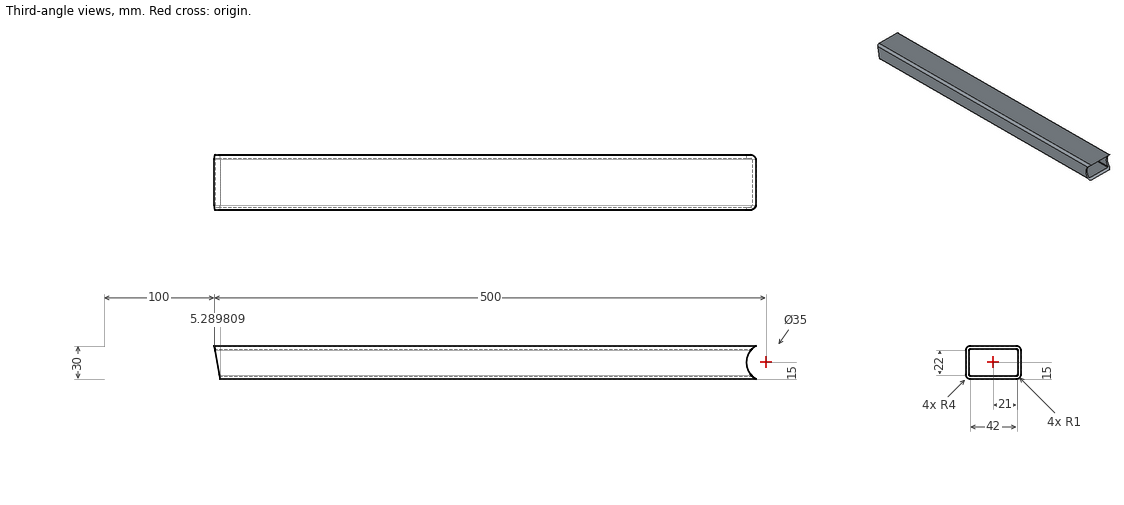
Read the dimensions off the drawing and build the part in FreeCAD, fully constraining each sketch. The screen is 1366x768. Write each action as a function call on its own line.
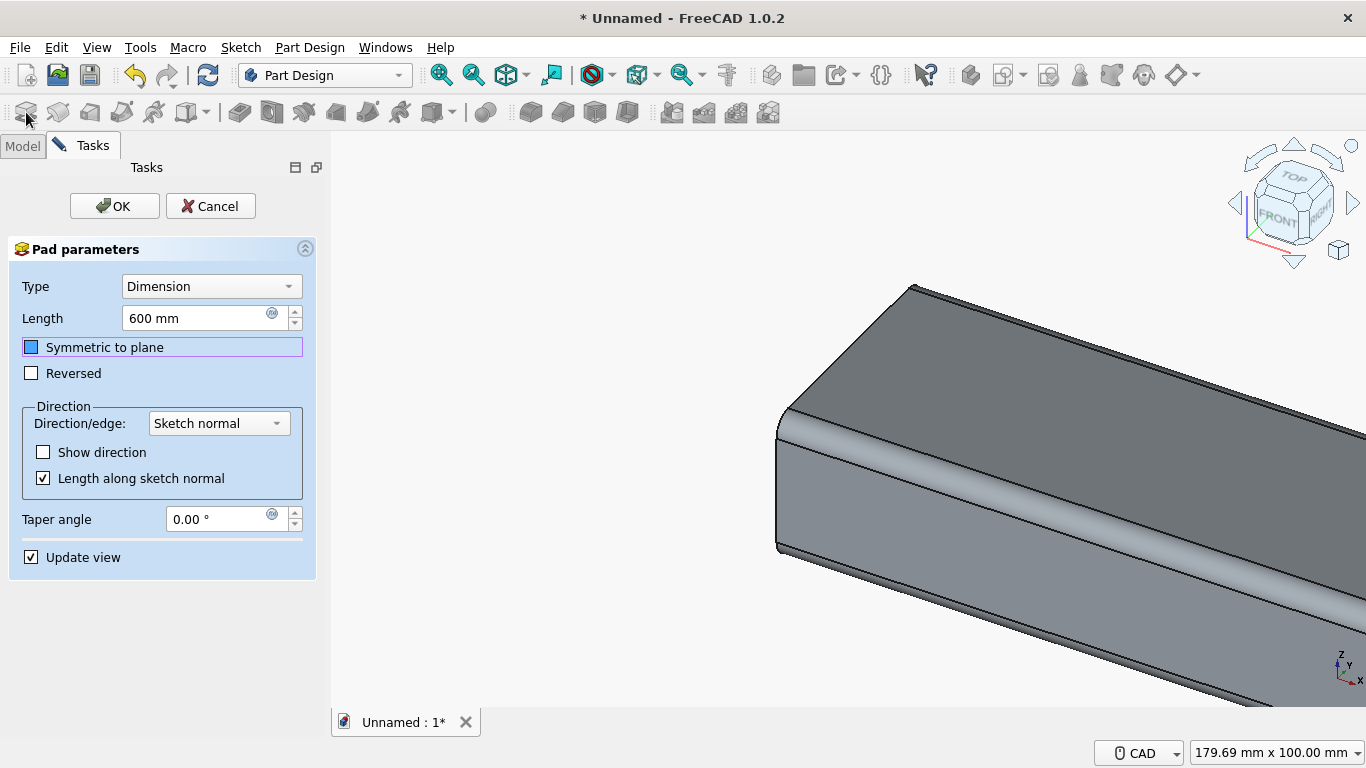
click(30, 373)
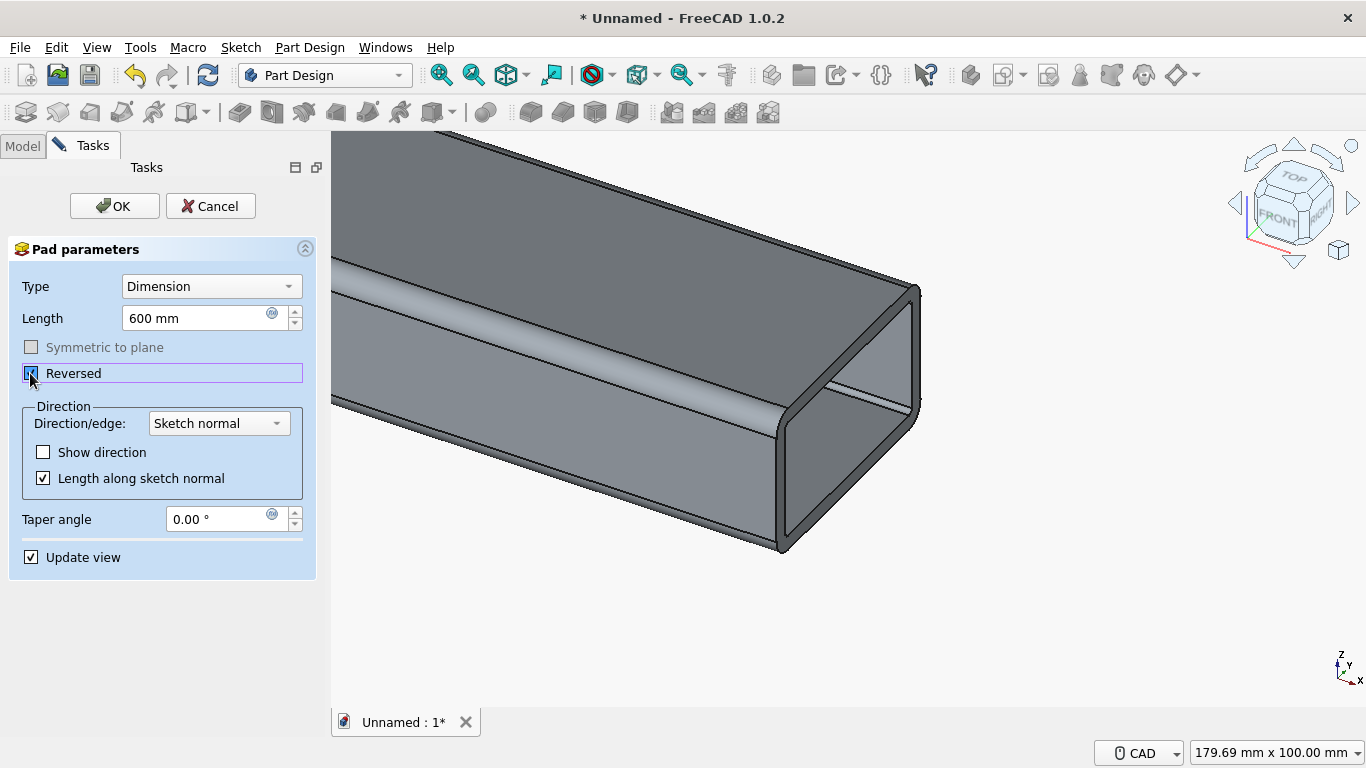
click(115, 206)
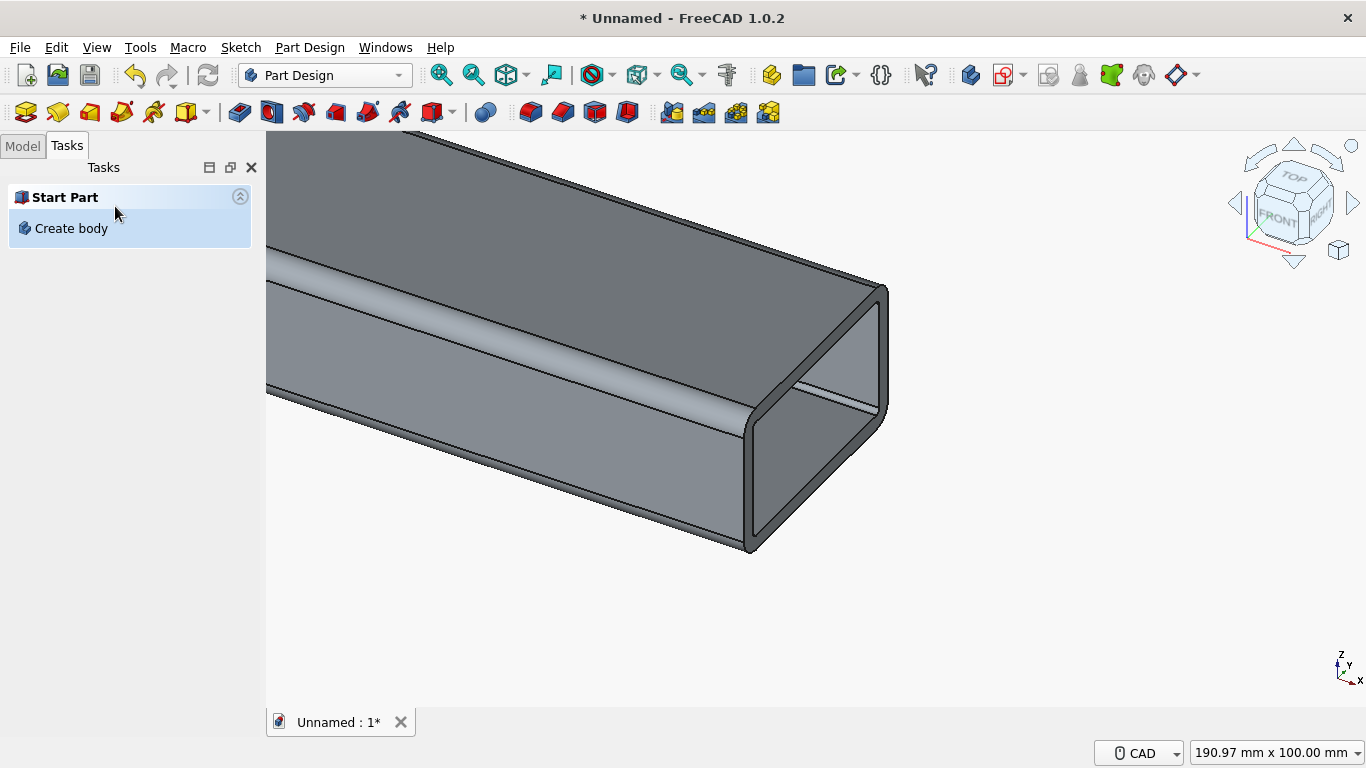
key(v)
key(f)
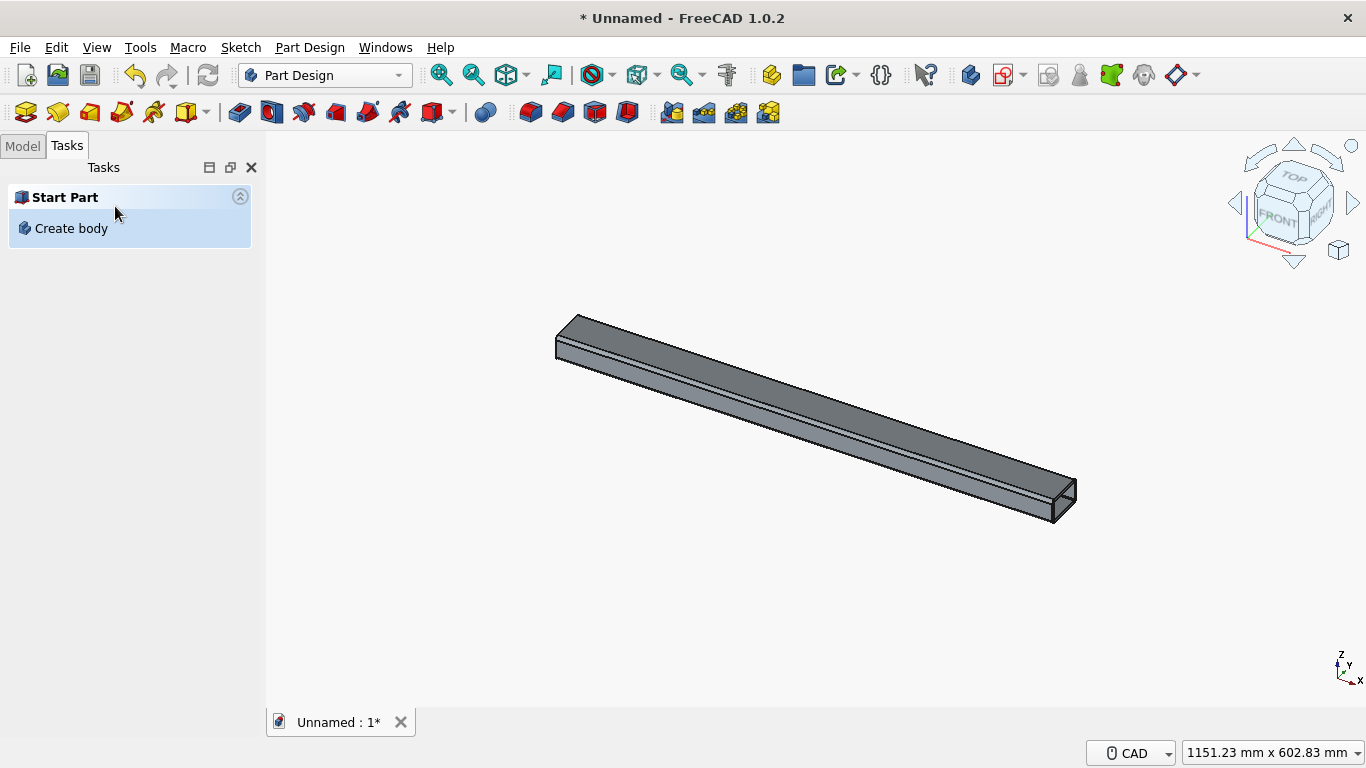
key(0)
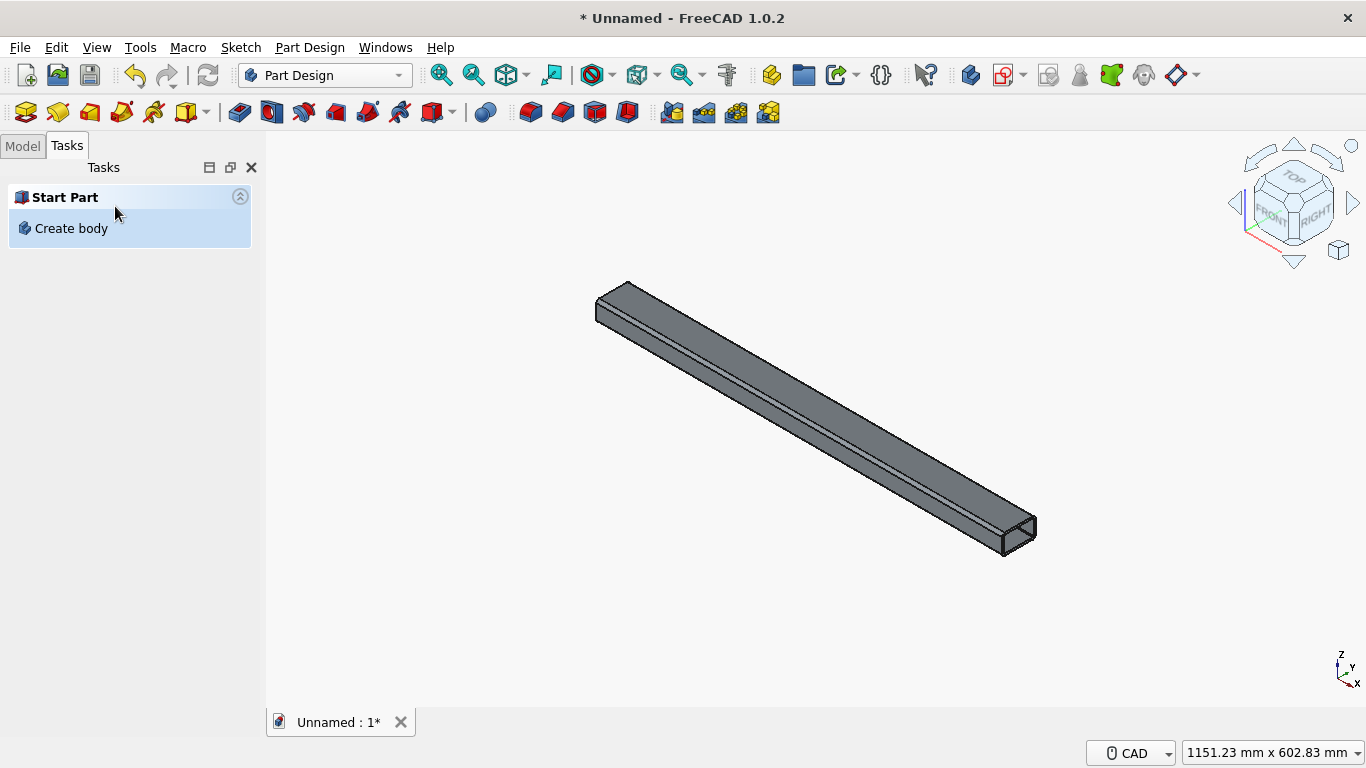
key(1)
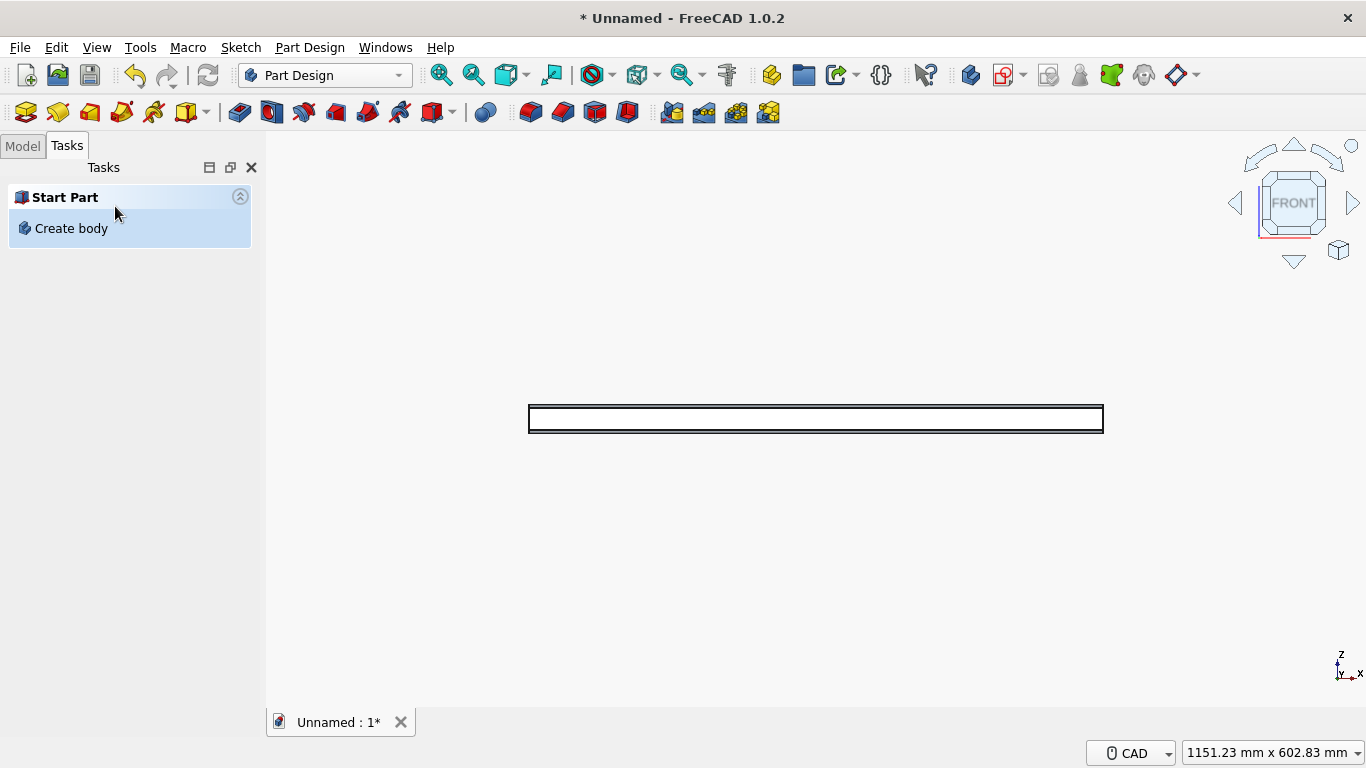
click(816, 418)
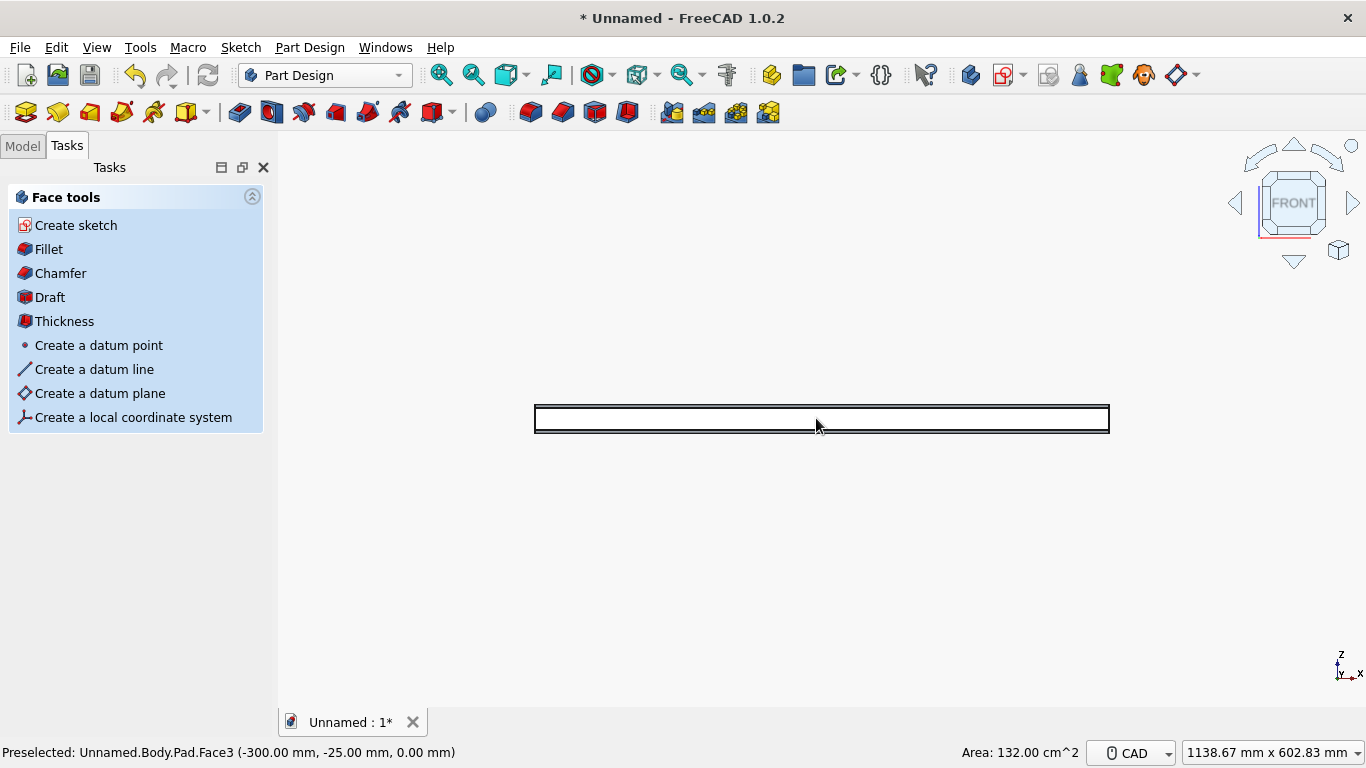
click(1004, 76)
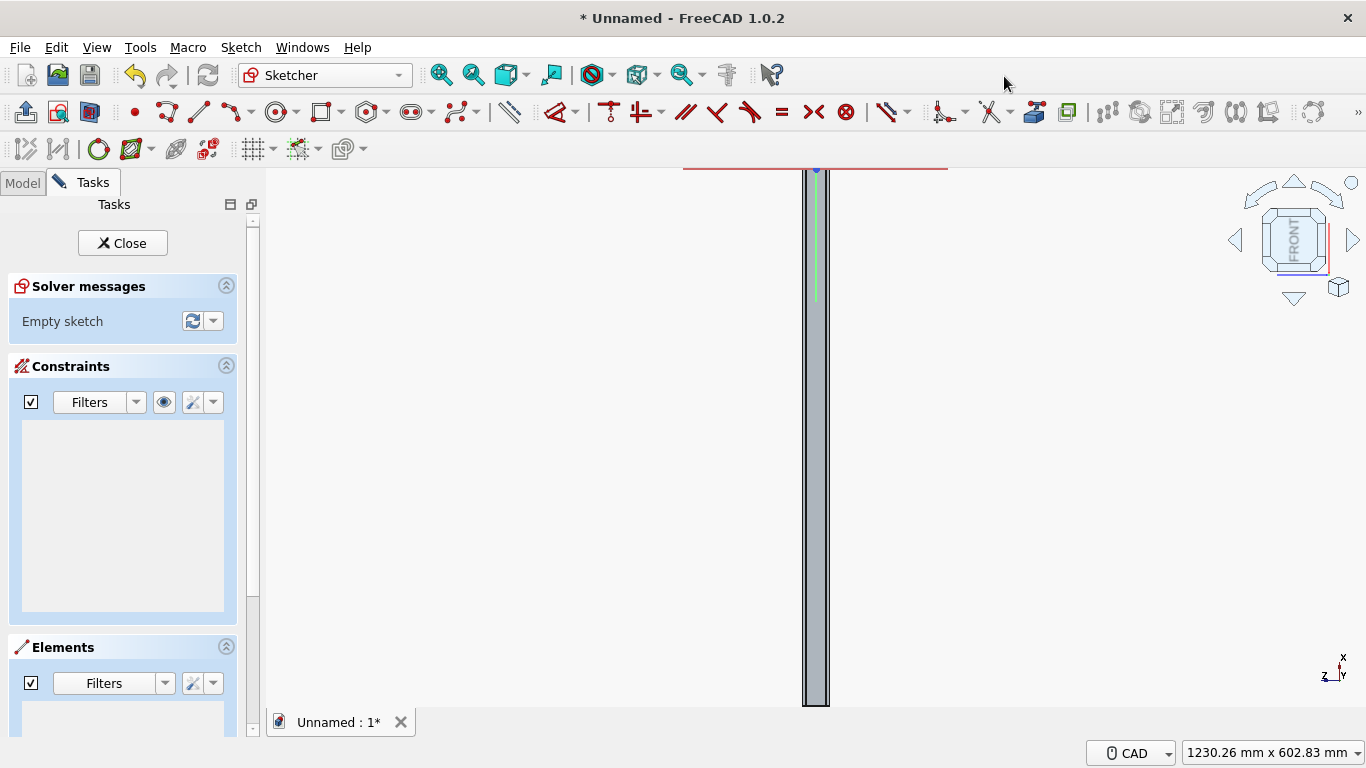
scroll(748, 438, down, 5)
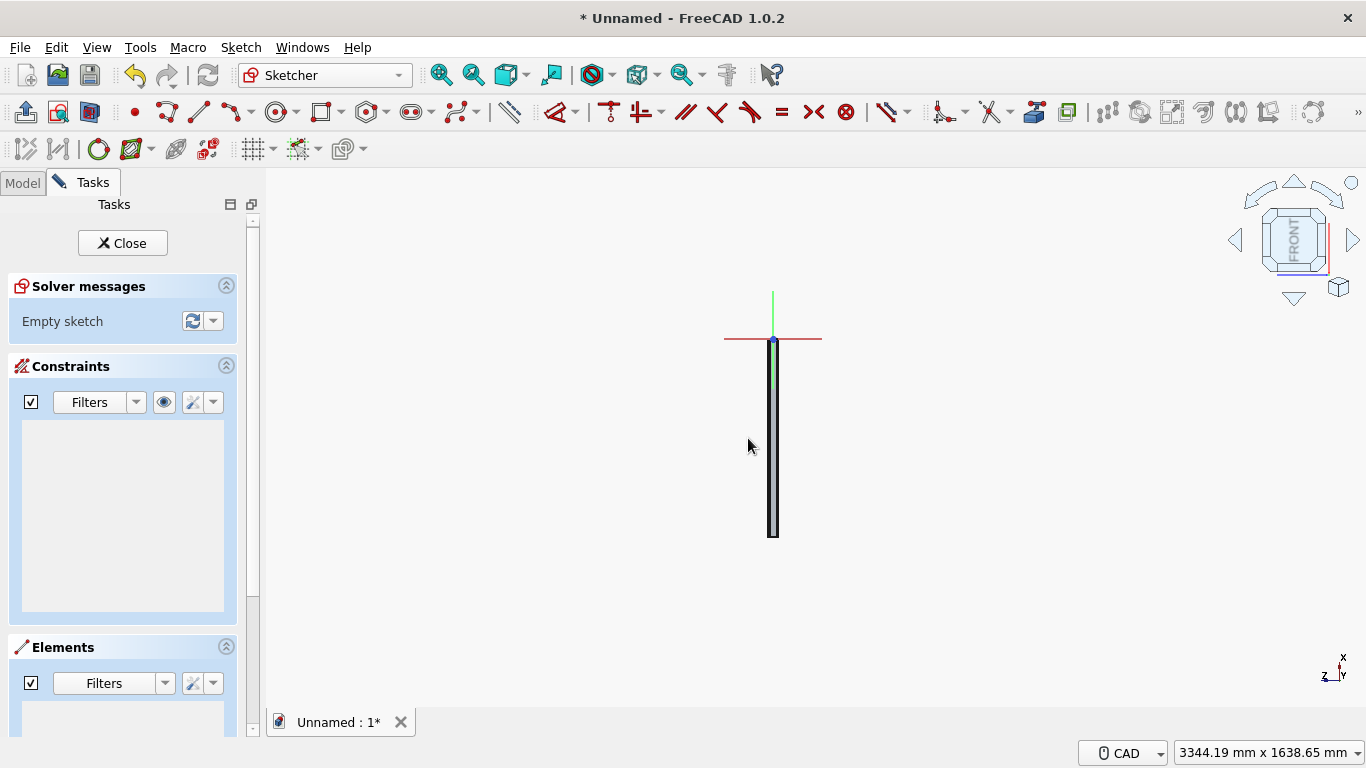
scroll(777, 530, up, 11)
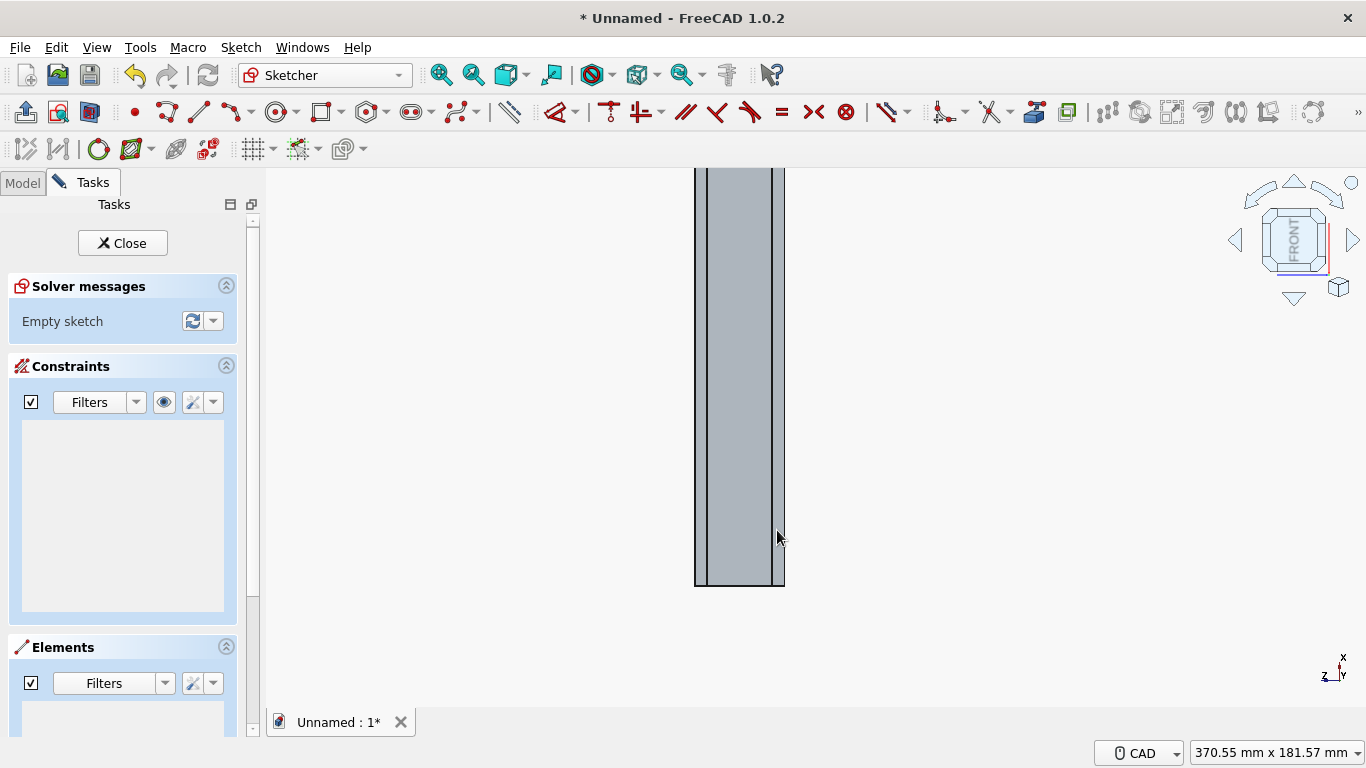
key(g)
key(m)